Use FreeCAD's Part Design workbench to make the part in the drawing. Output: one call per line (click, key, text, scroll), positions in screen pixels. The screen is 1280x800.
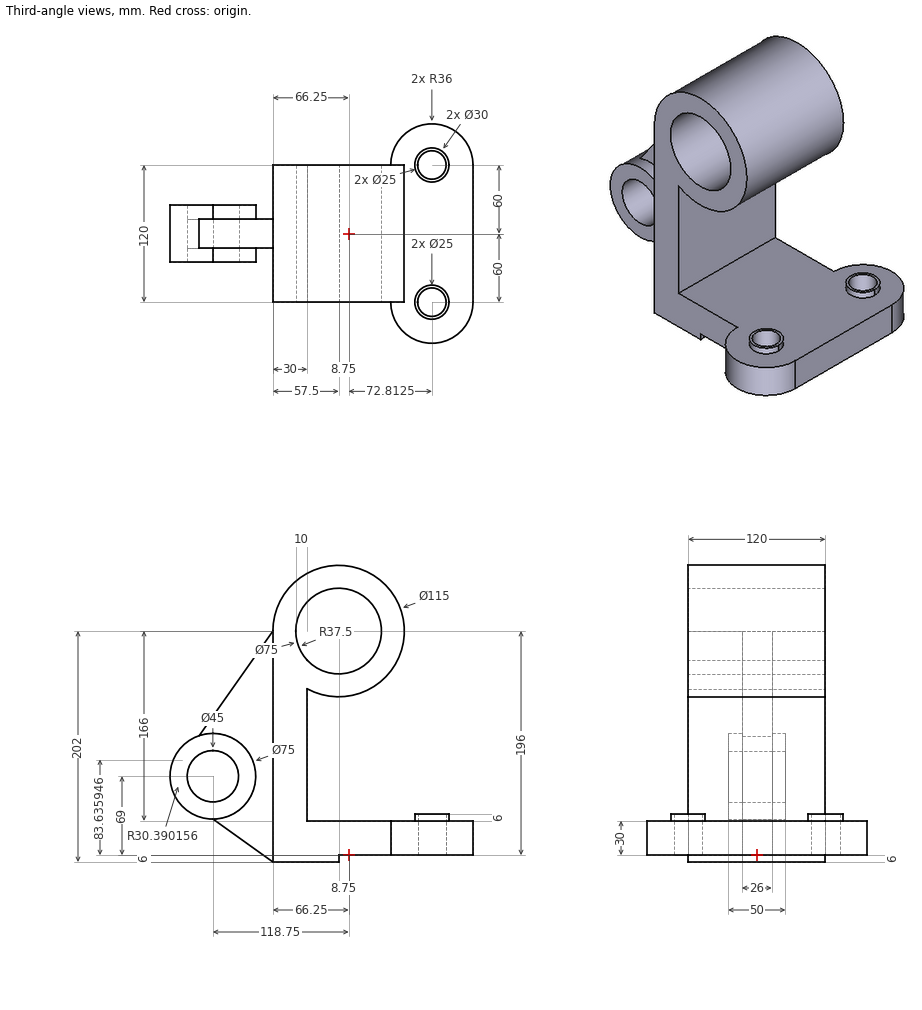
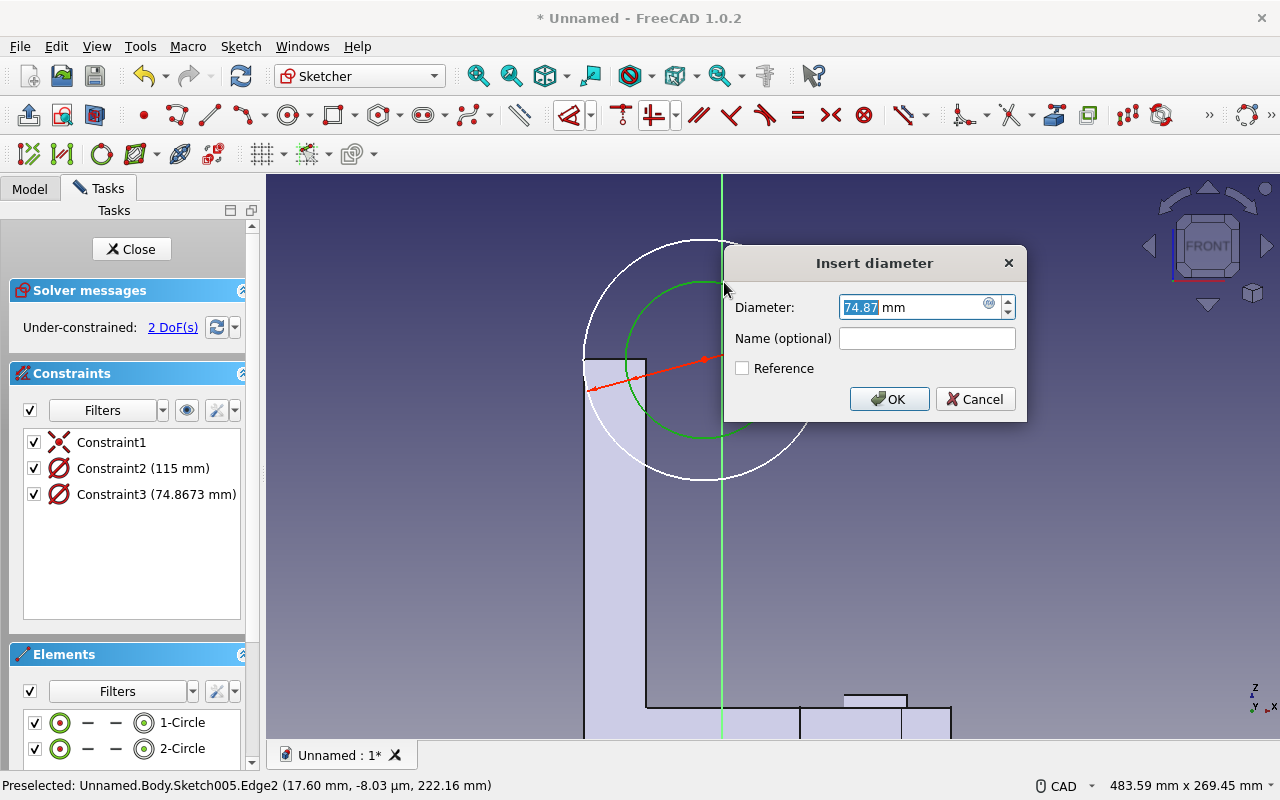
text(75)
key(Return)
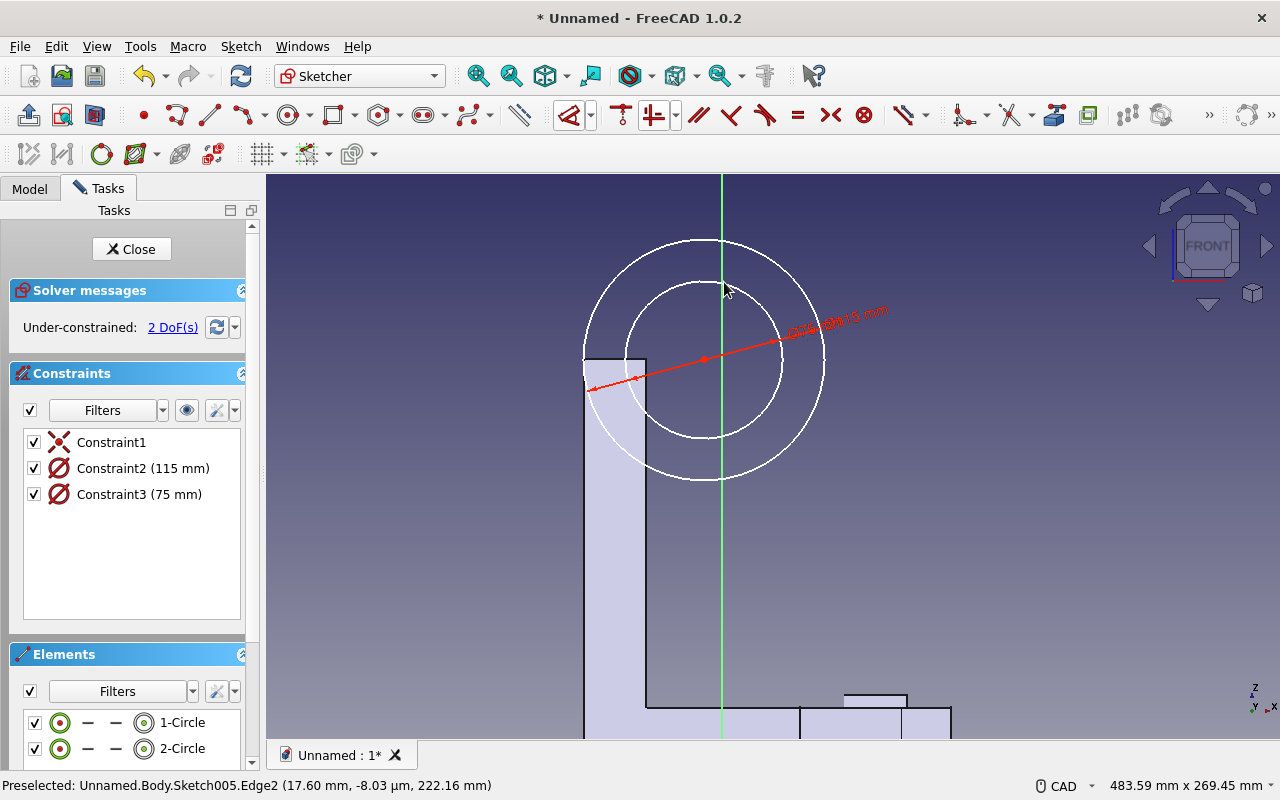
click(704, 360)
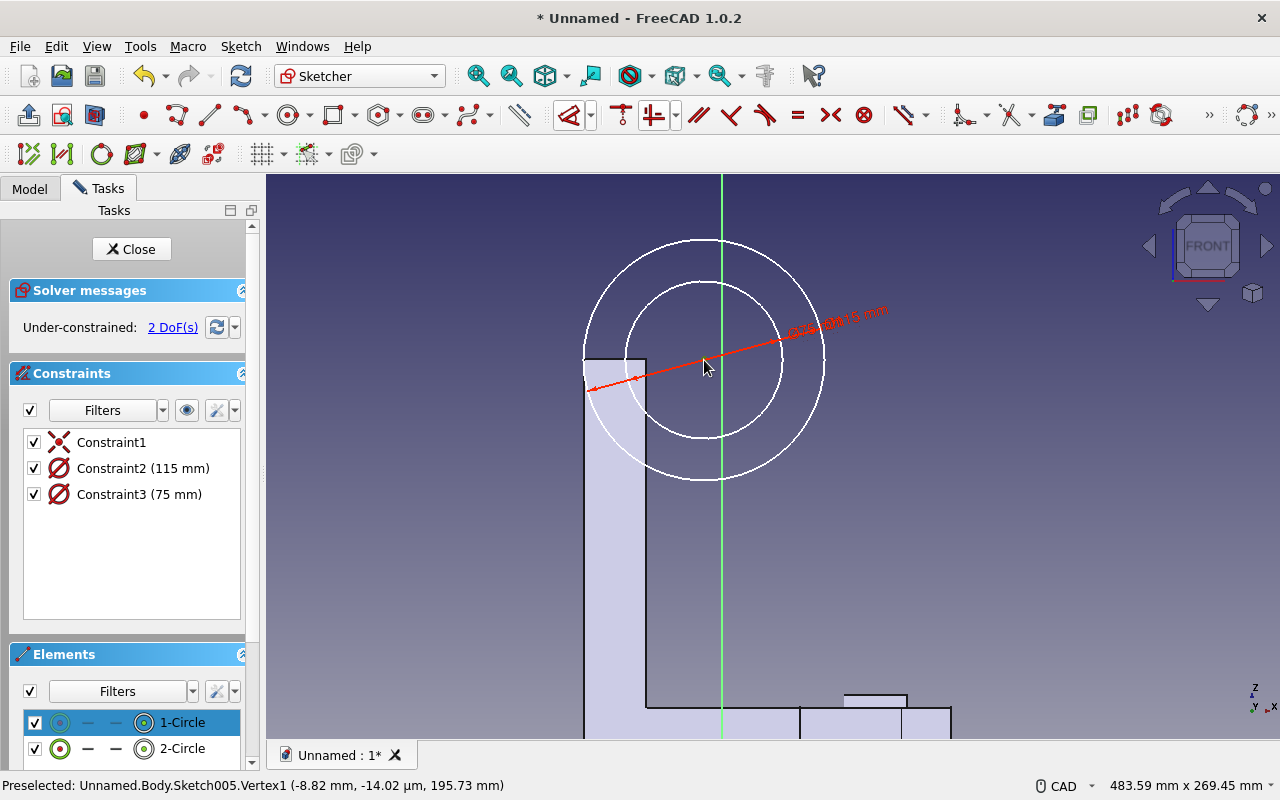
key(i)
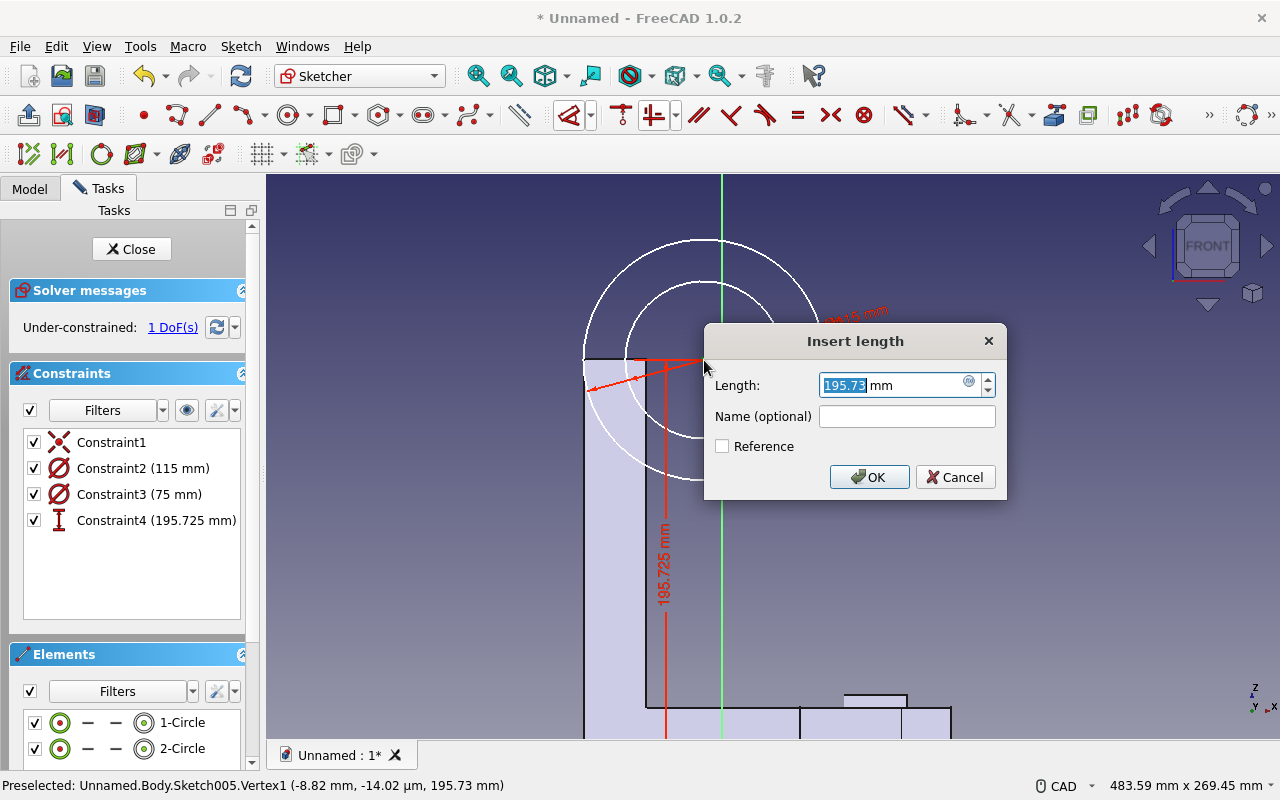
text(196)
key(Return)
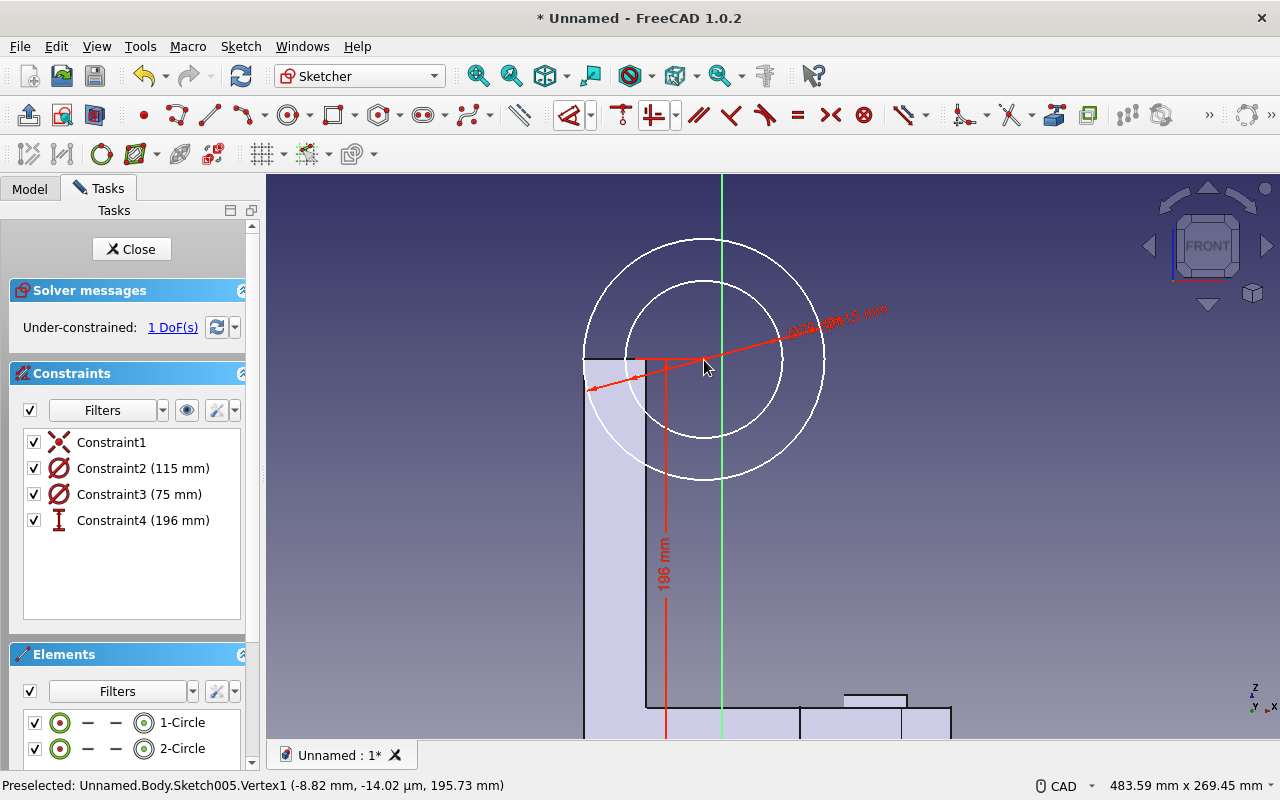
scroll(704, 359, up, 4)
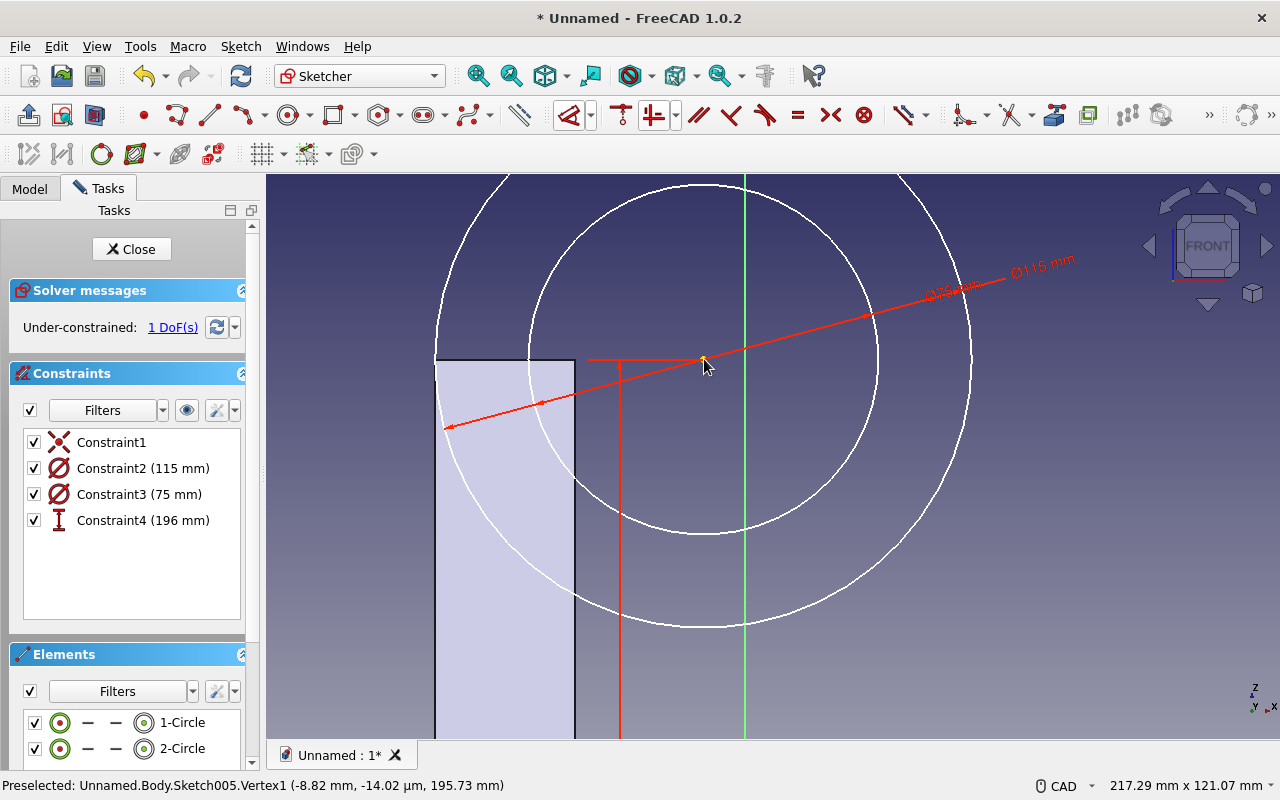
click(703, 360)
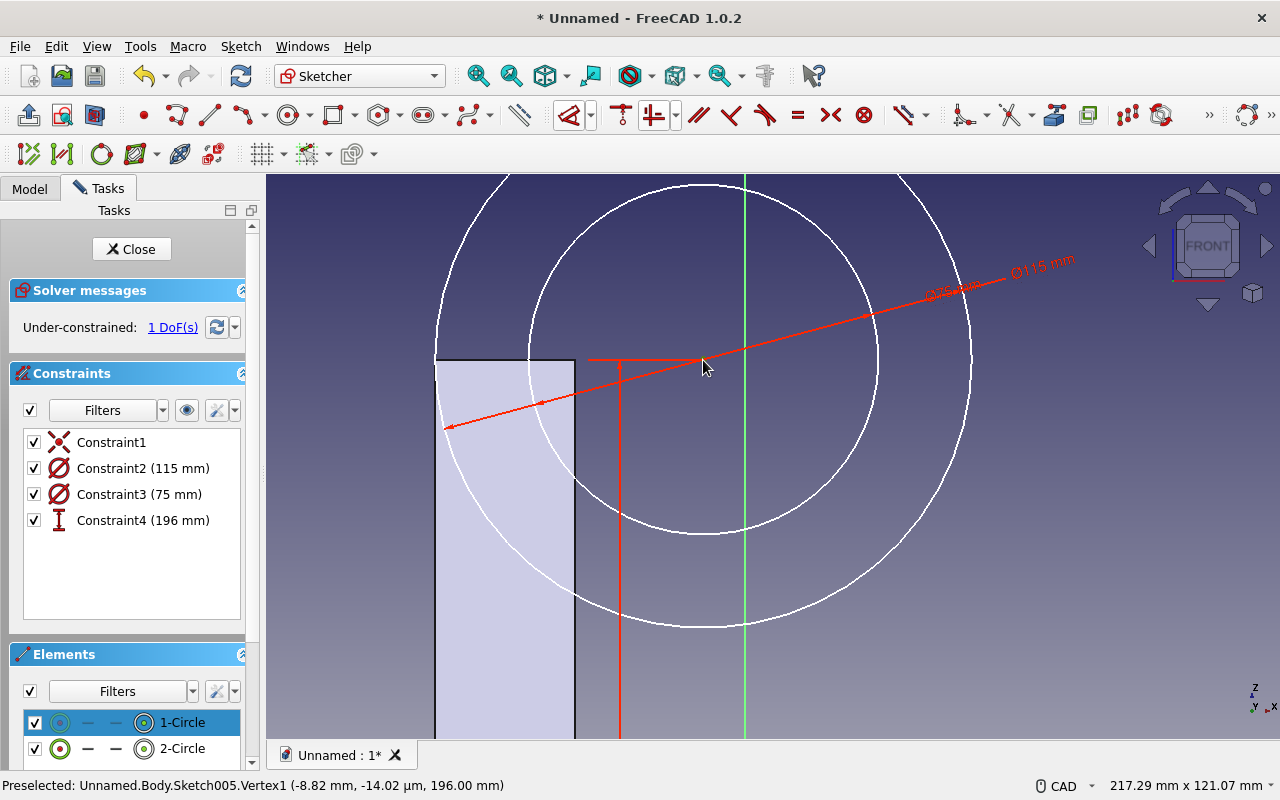
key(l)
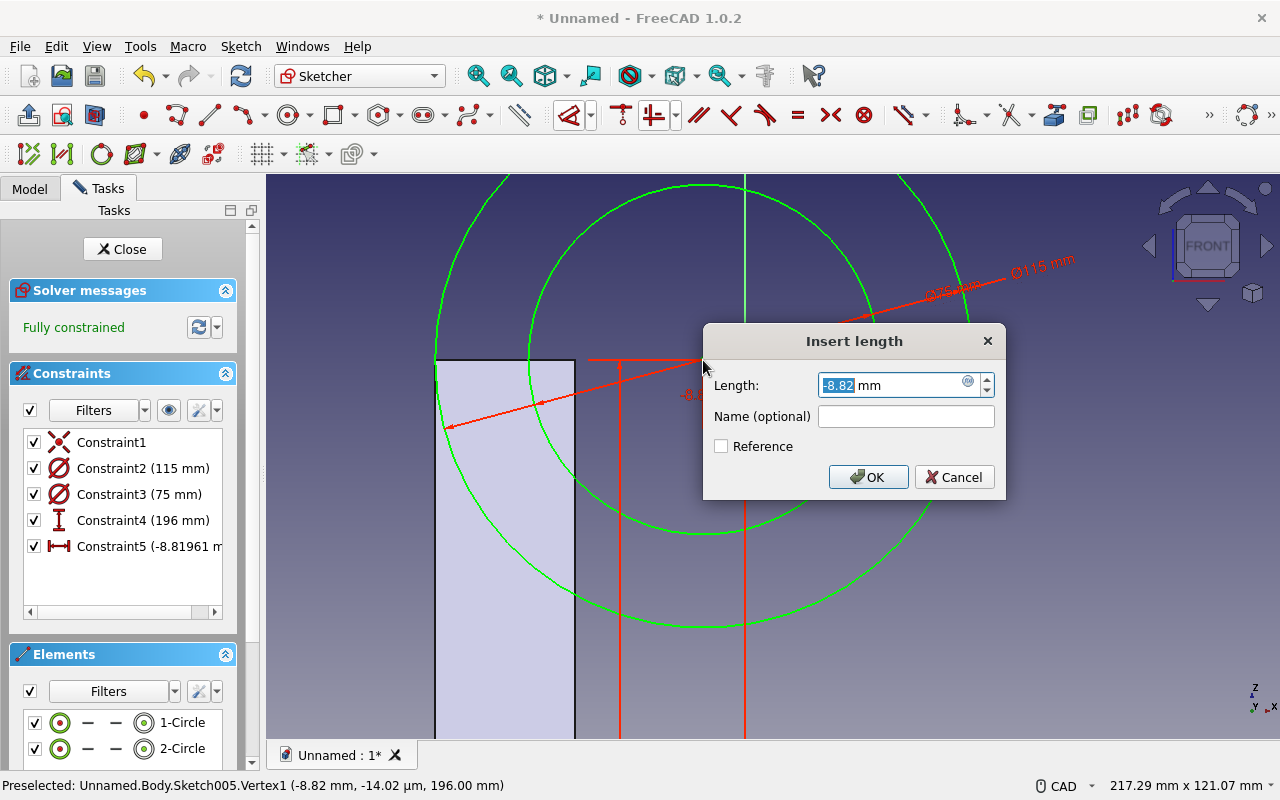
text(-8.75)
key(Return)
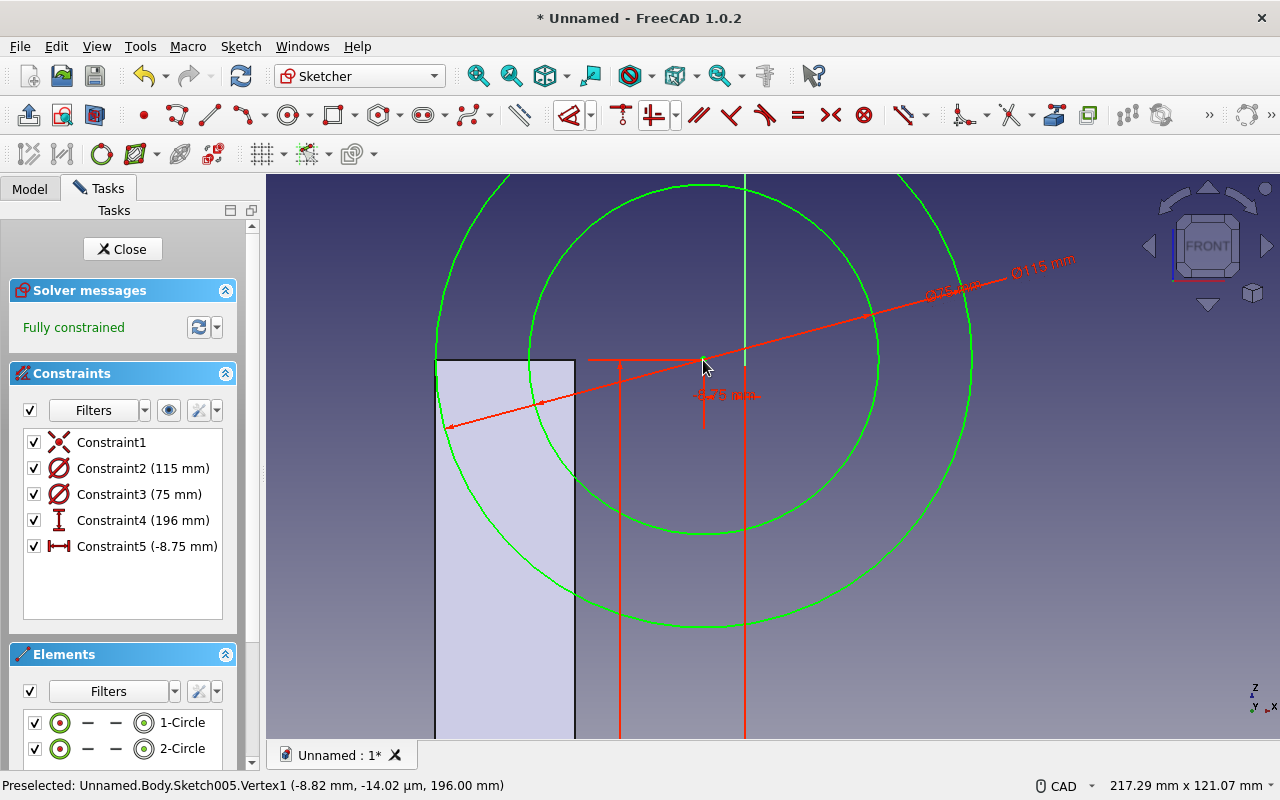
click(123, 249)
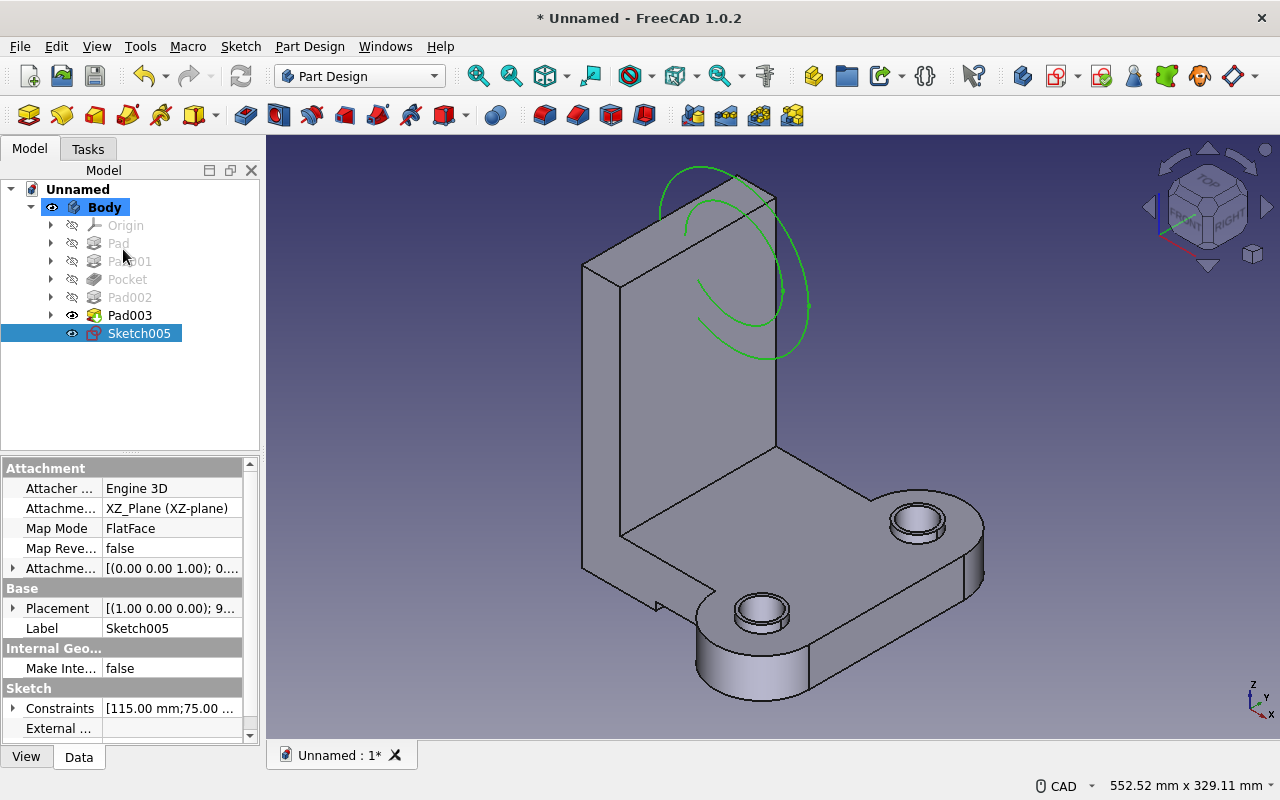
click(29, 116)